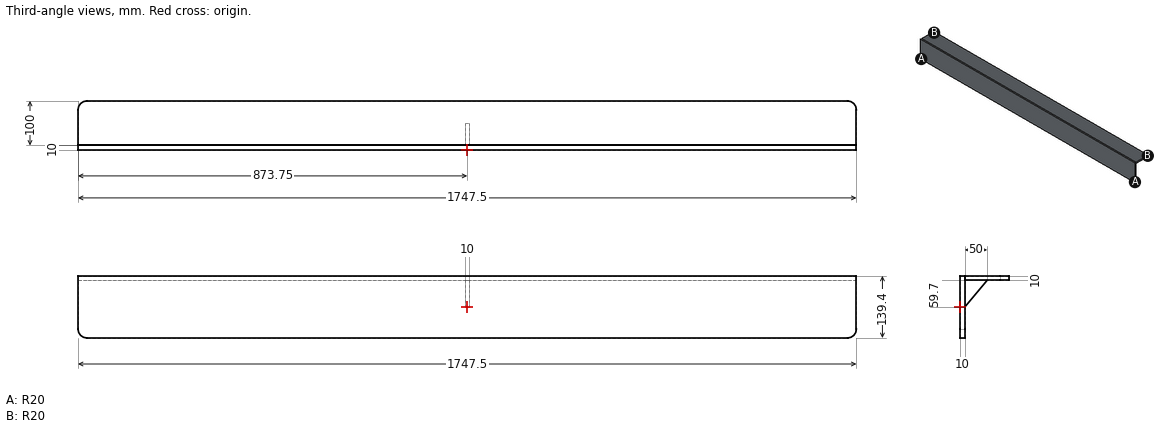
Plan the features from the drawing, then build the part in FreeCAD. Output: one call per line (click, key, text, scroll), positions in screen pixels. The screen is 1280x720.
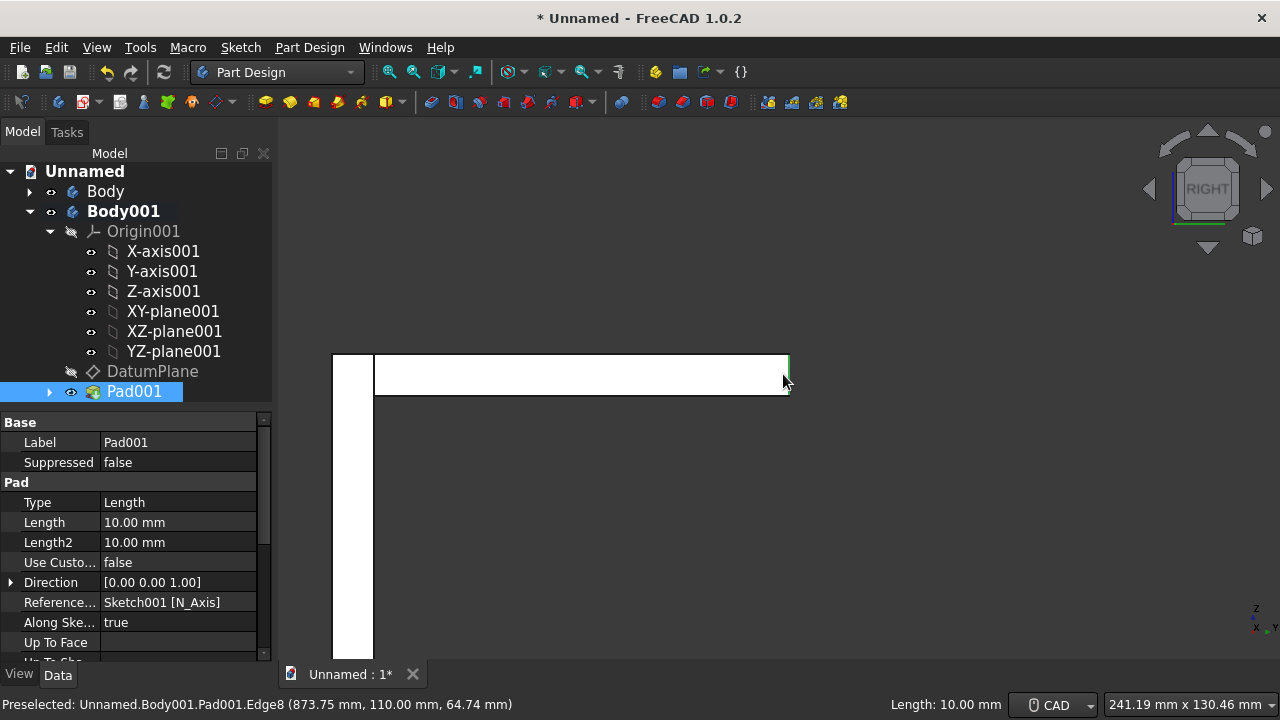
click(390, 72)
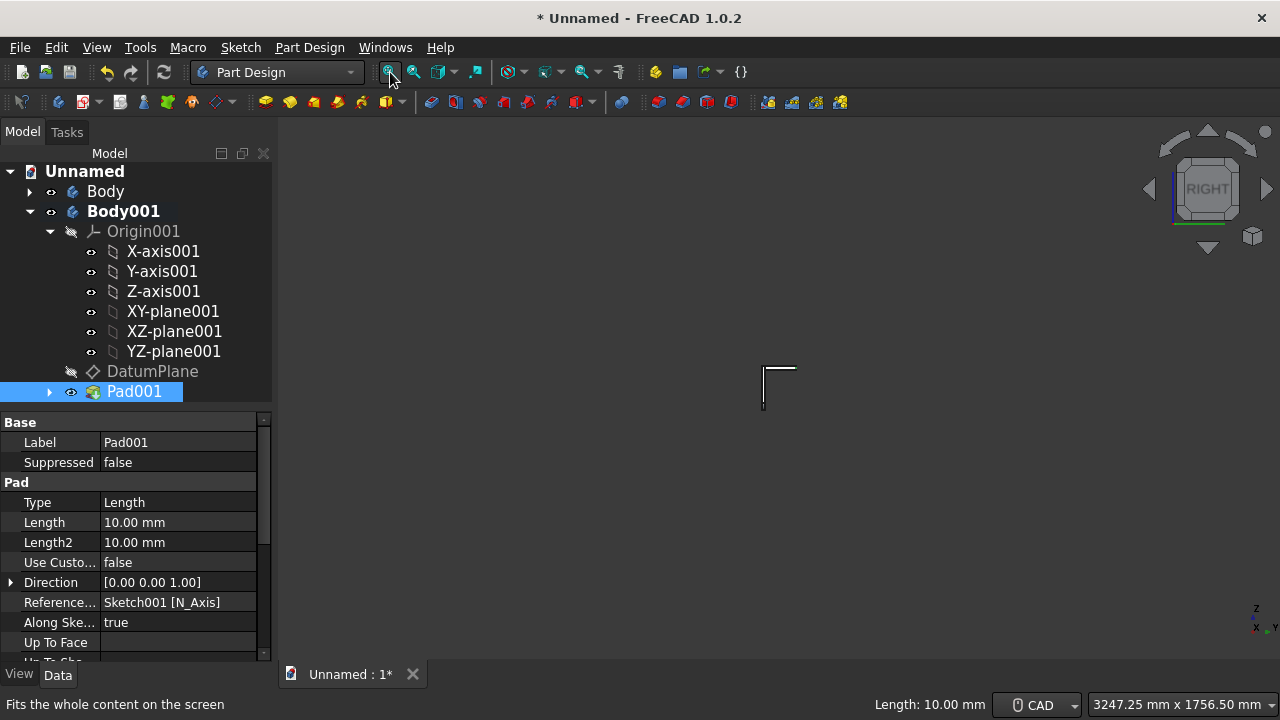
key(5)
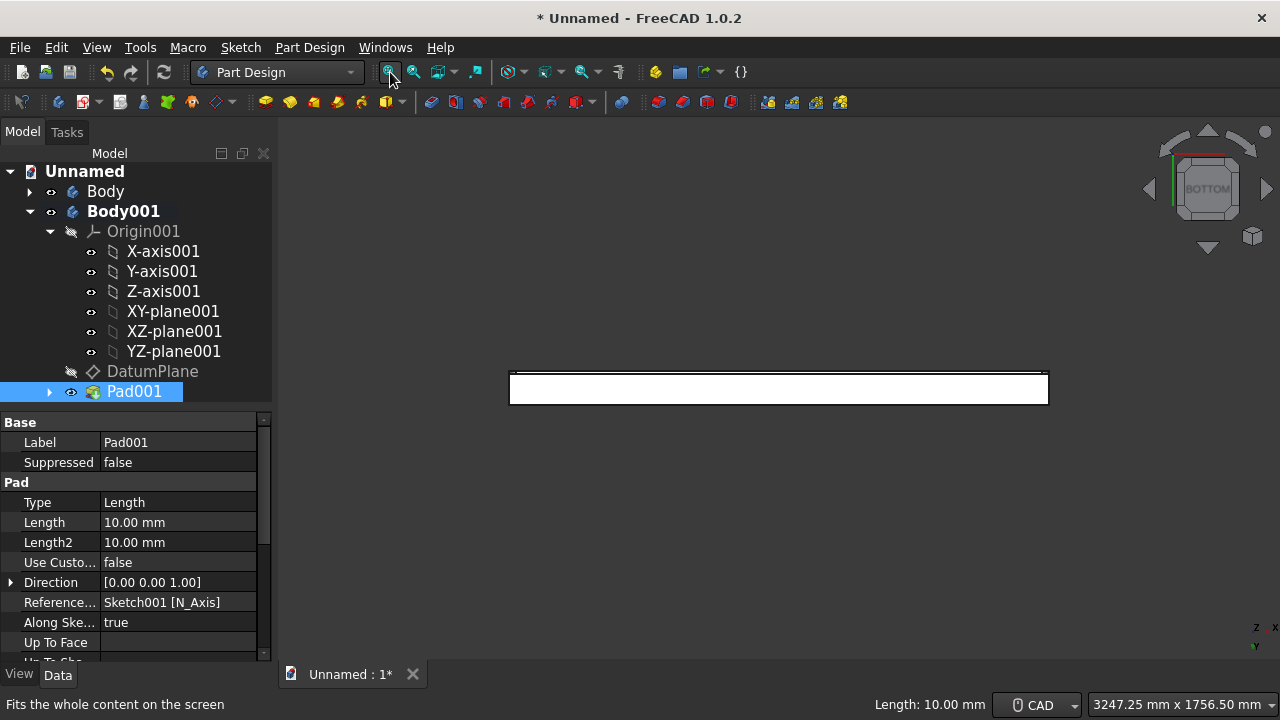
scroll(509, 404, up, 13)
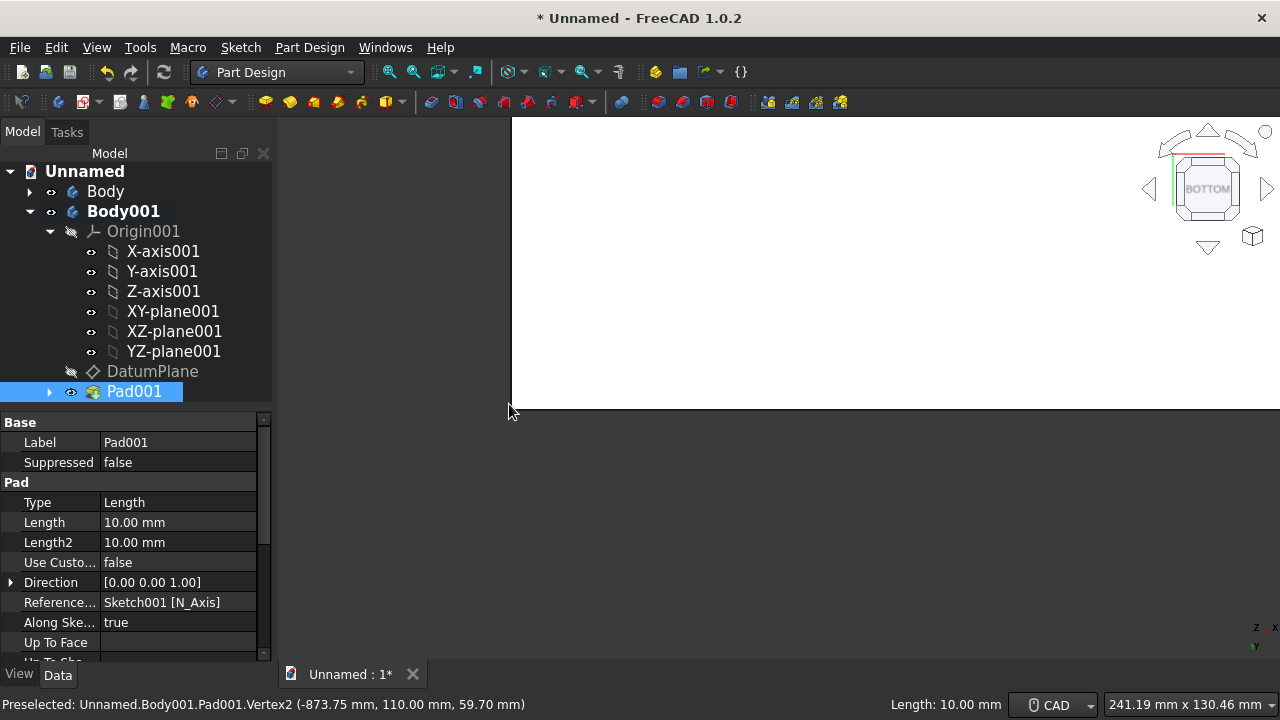
click(390, 72)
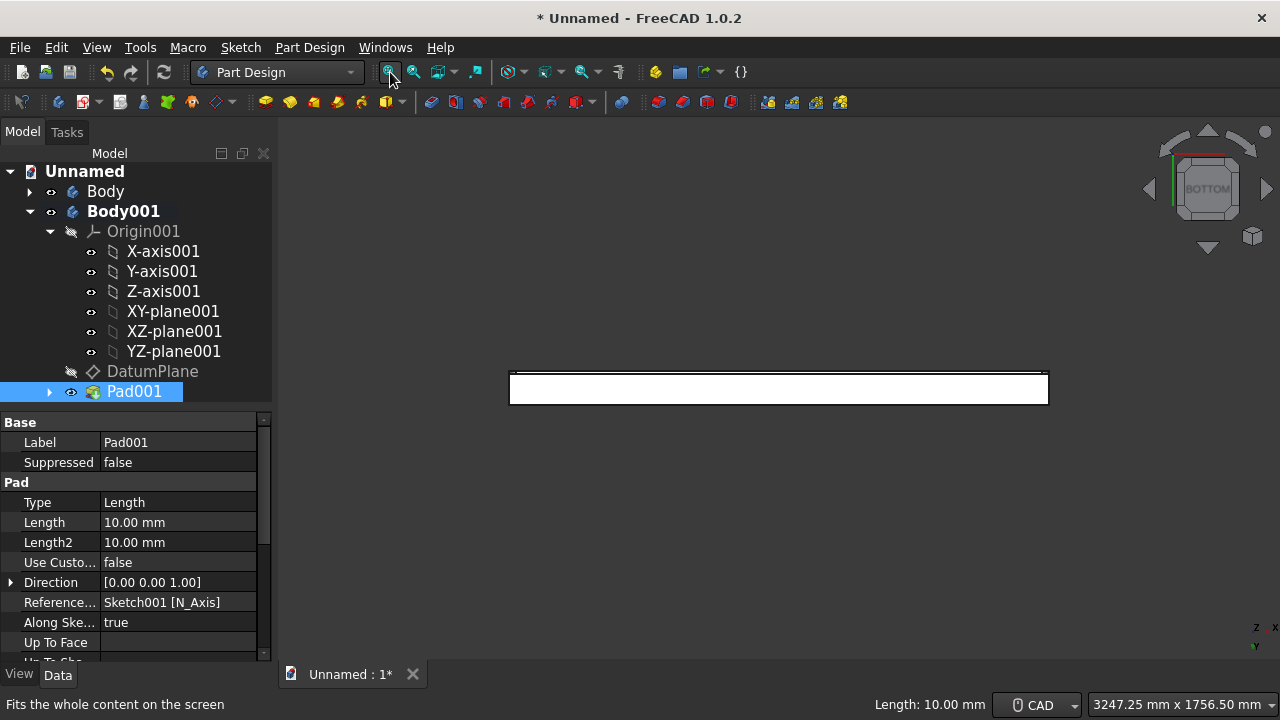
key(4)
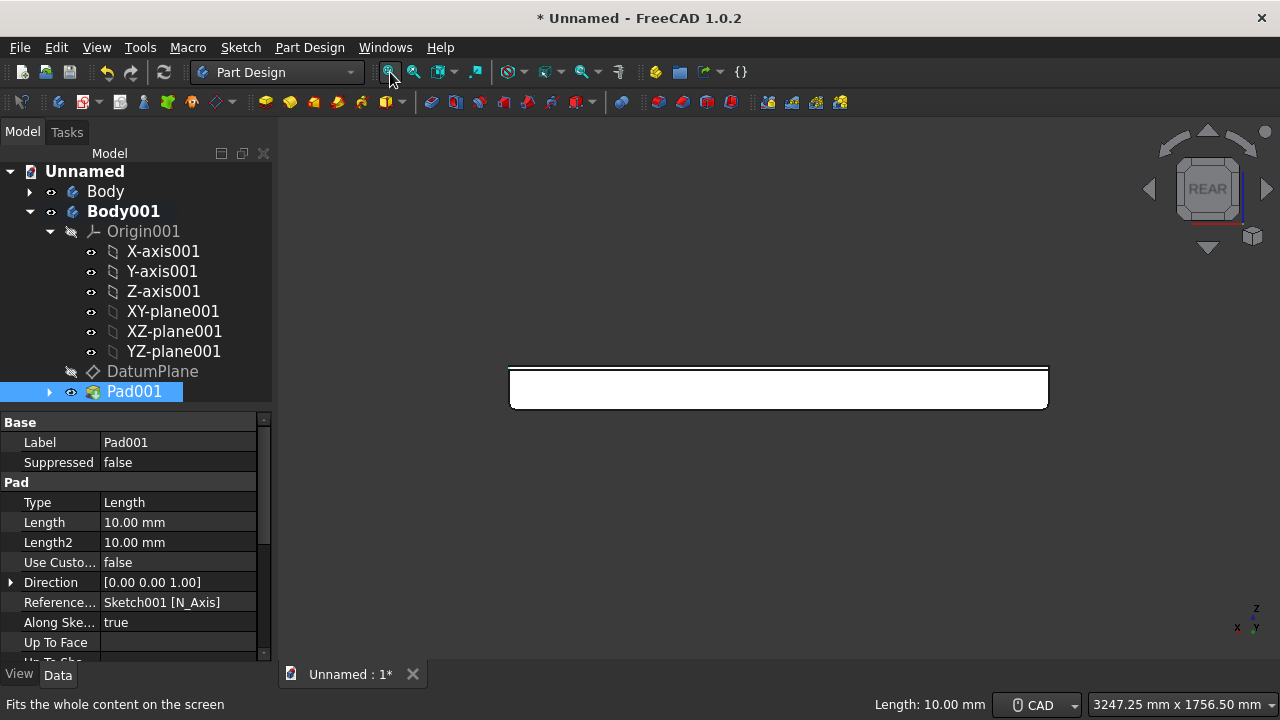
scroll(1049, 367, up, 13)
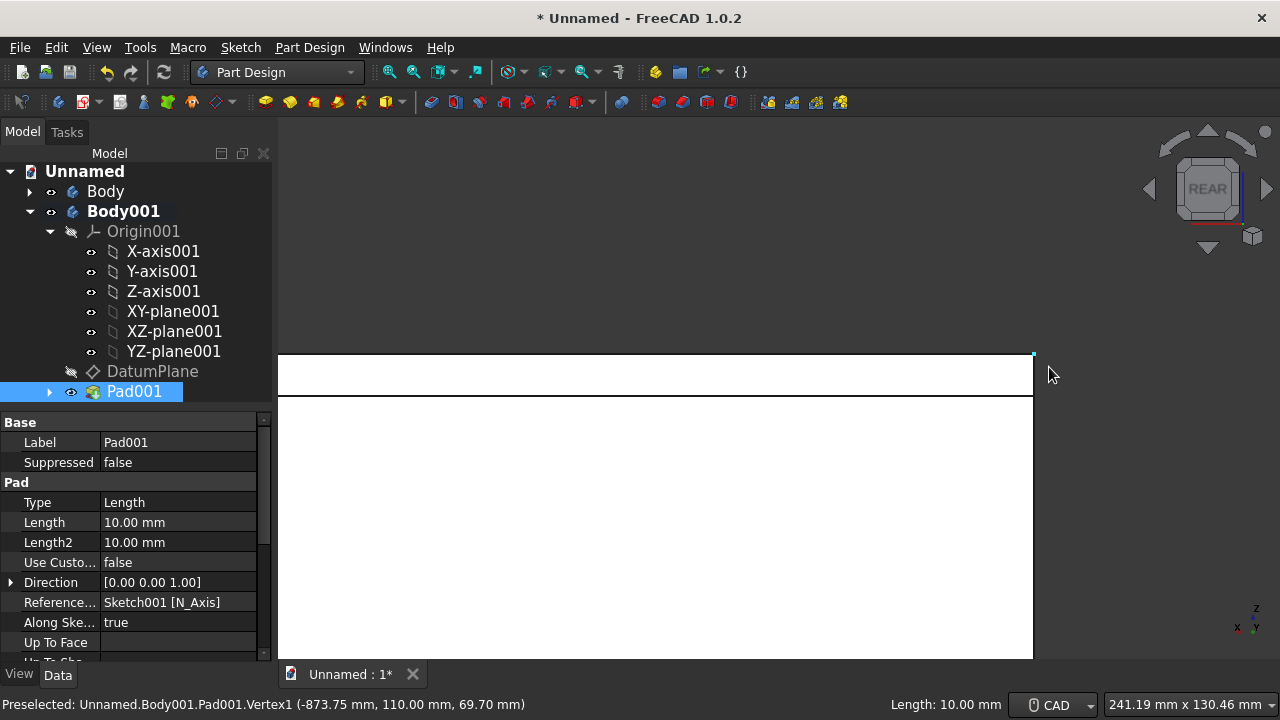
click(1034, 374, ctrl)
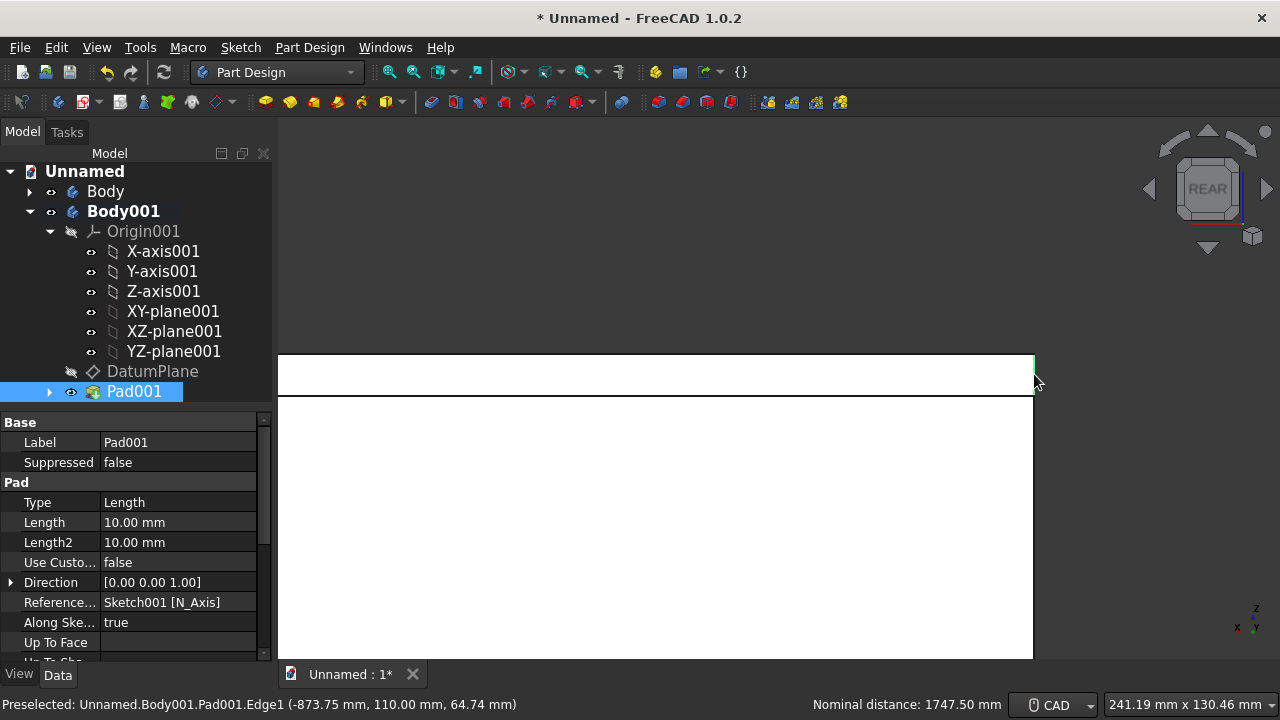
click(660, 102)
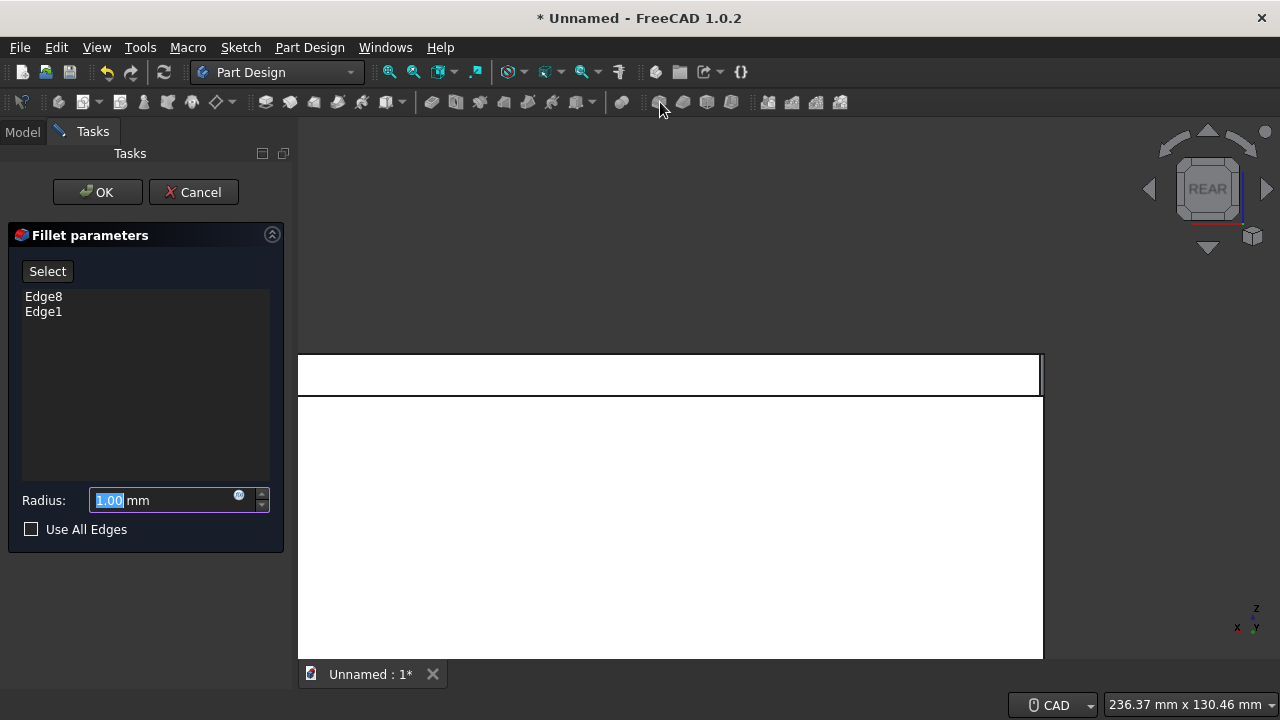
text(20)
key(Tab)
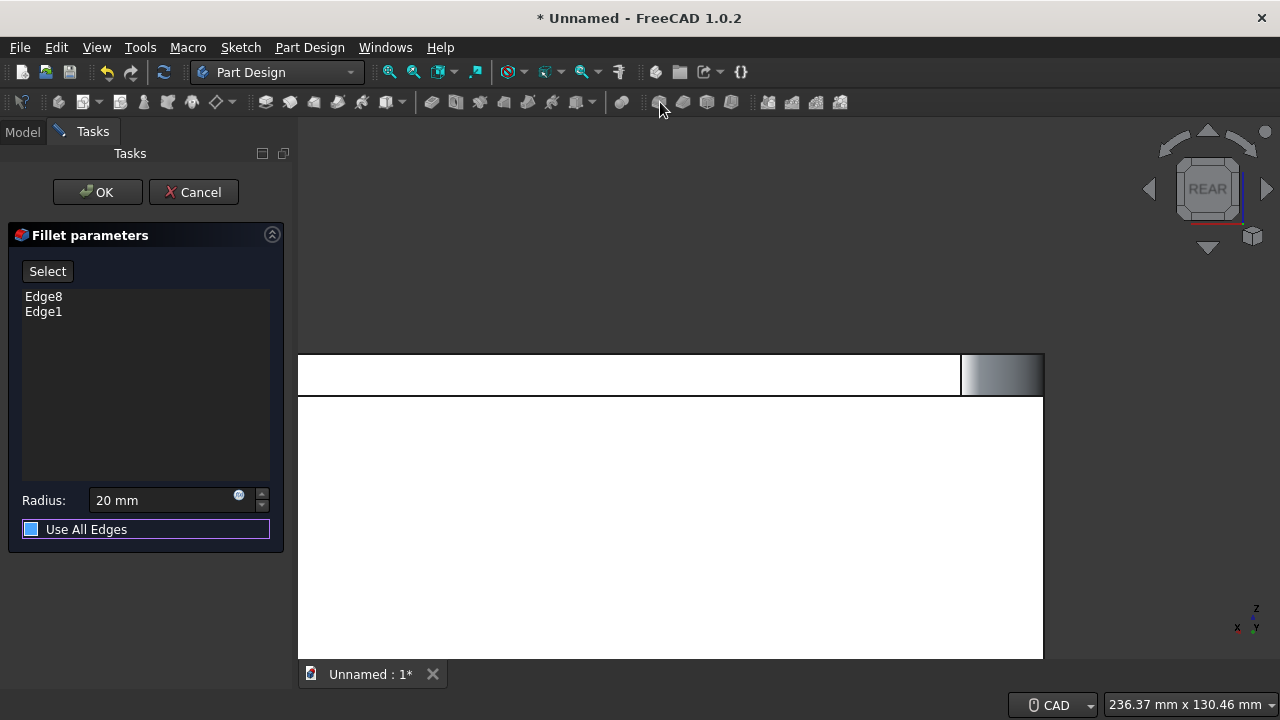
click(98, 192)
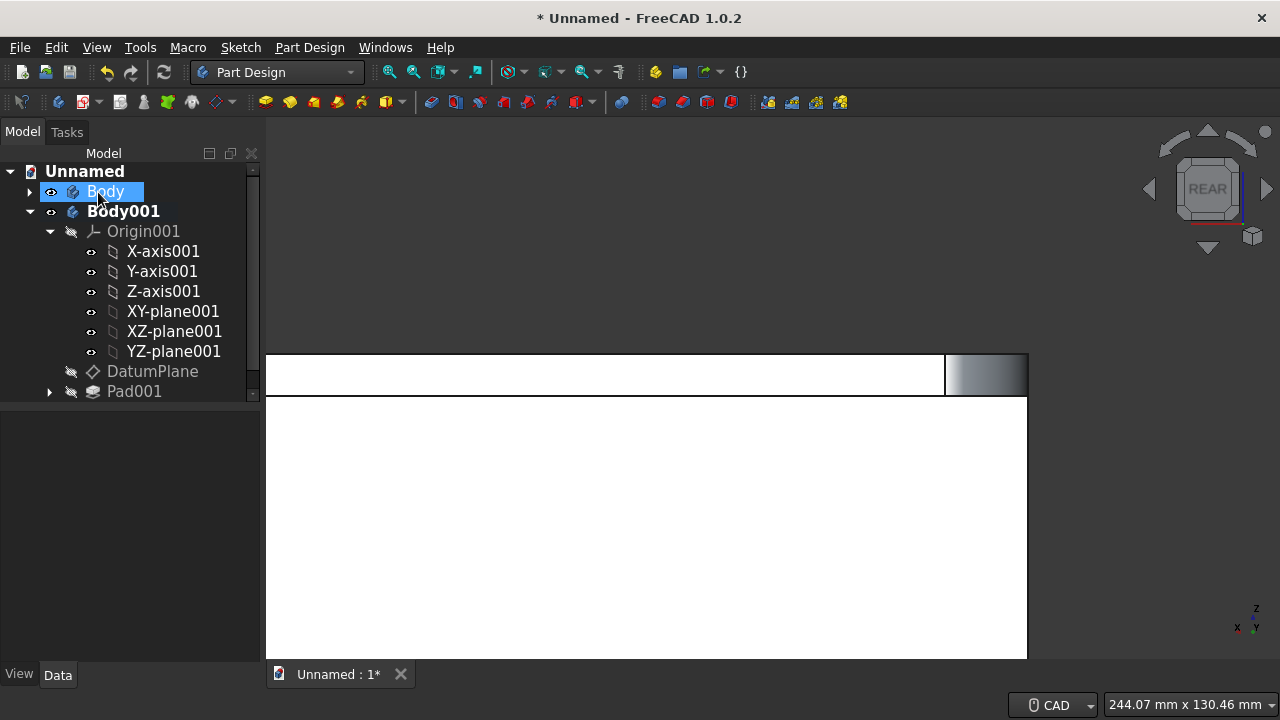
click(390, 72)